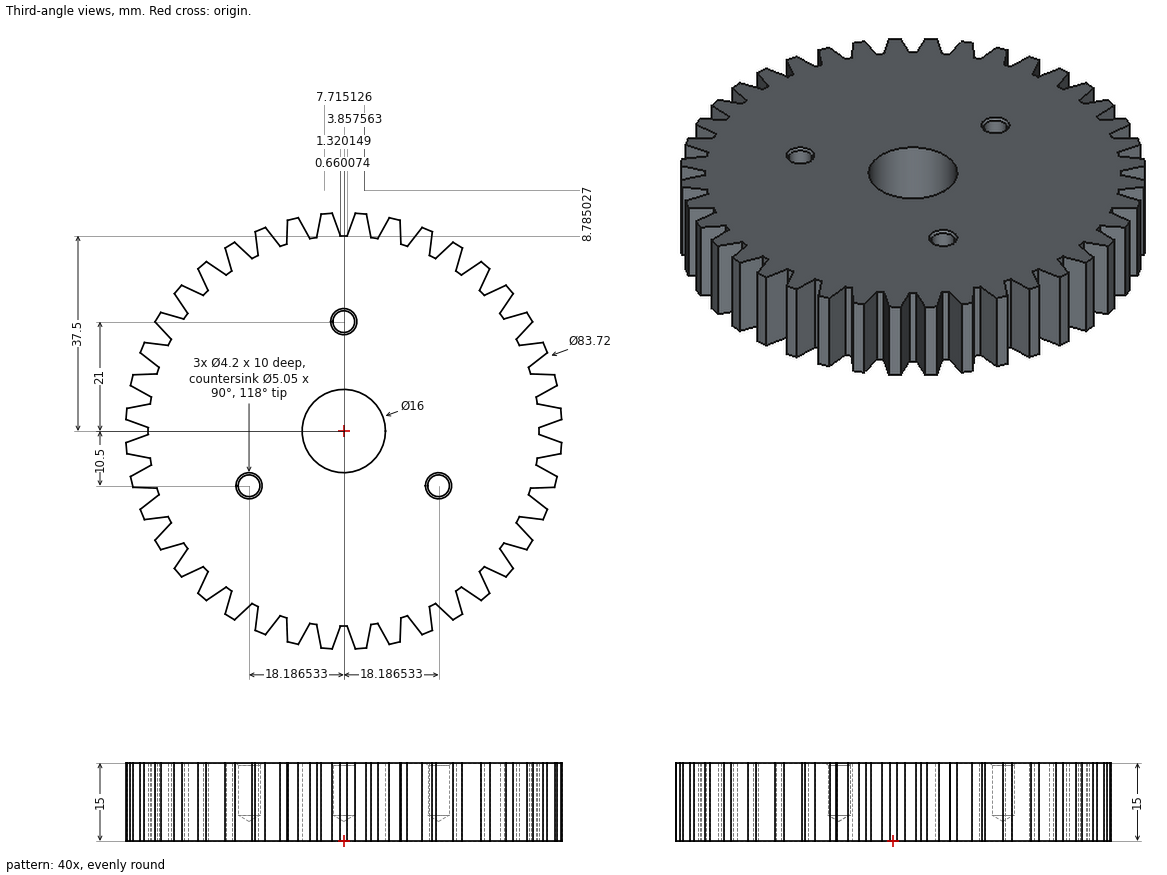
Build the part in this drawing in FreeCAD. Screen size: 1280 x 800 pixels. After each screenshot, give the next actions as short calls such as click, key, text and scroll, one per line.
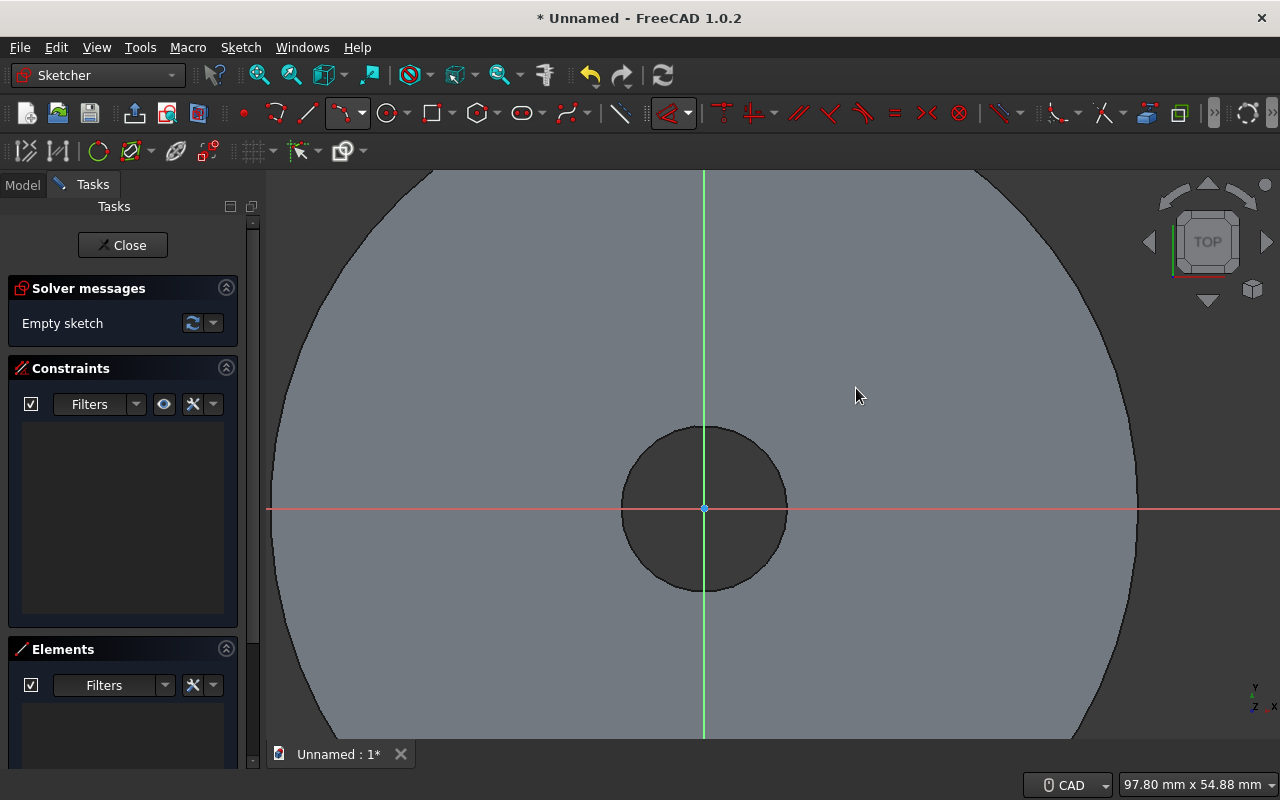
click(388, 114)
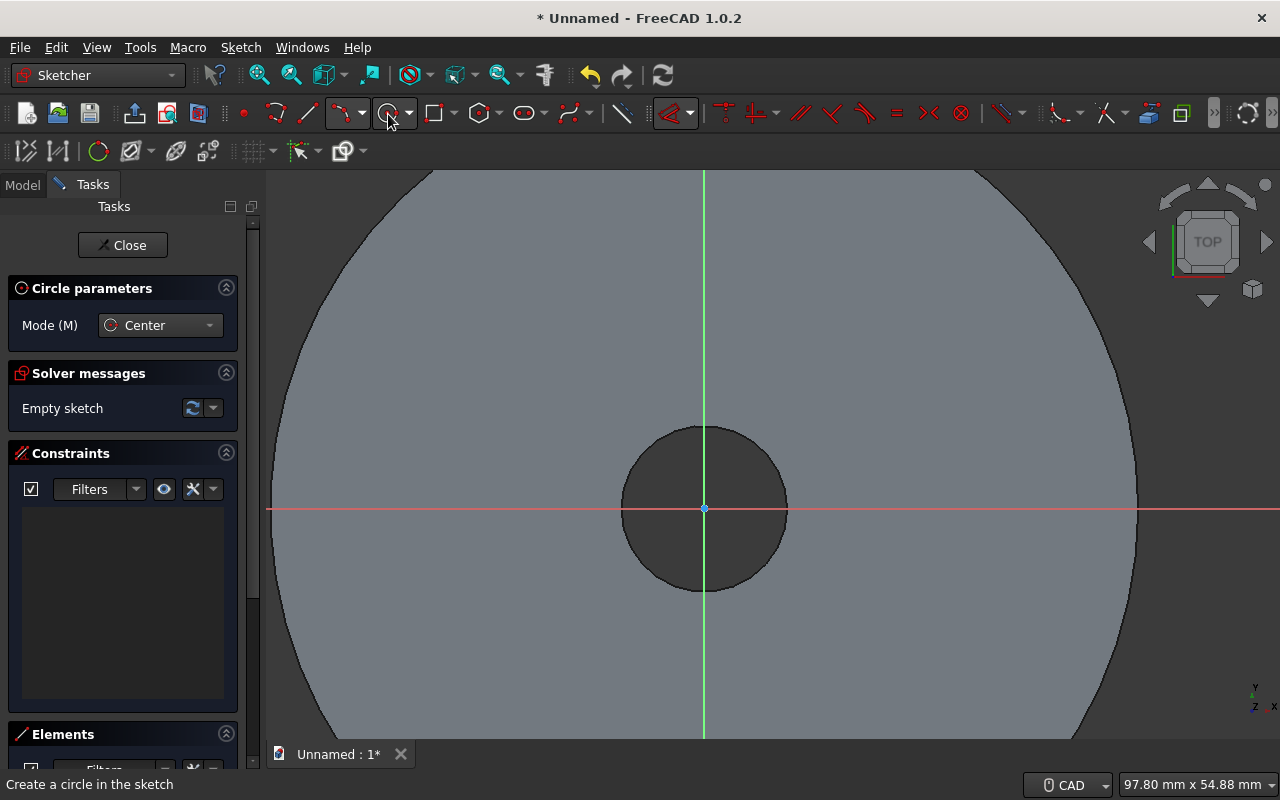
click(516, 618)
click(531, 602)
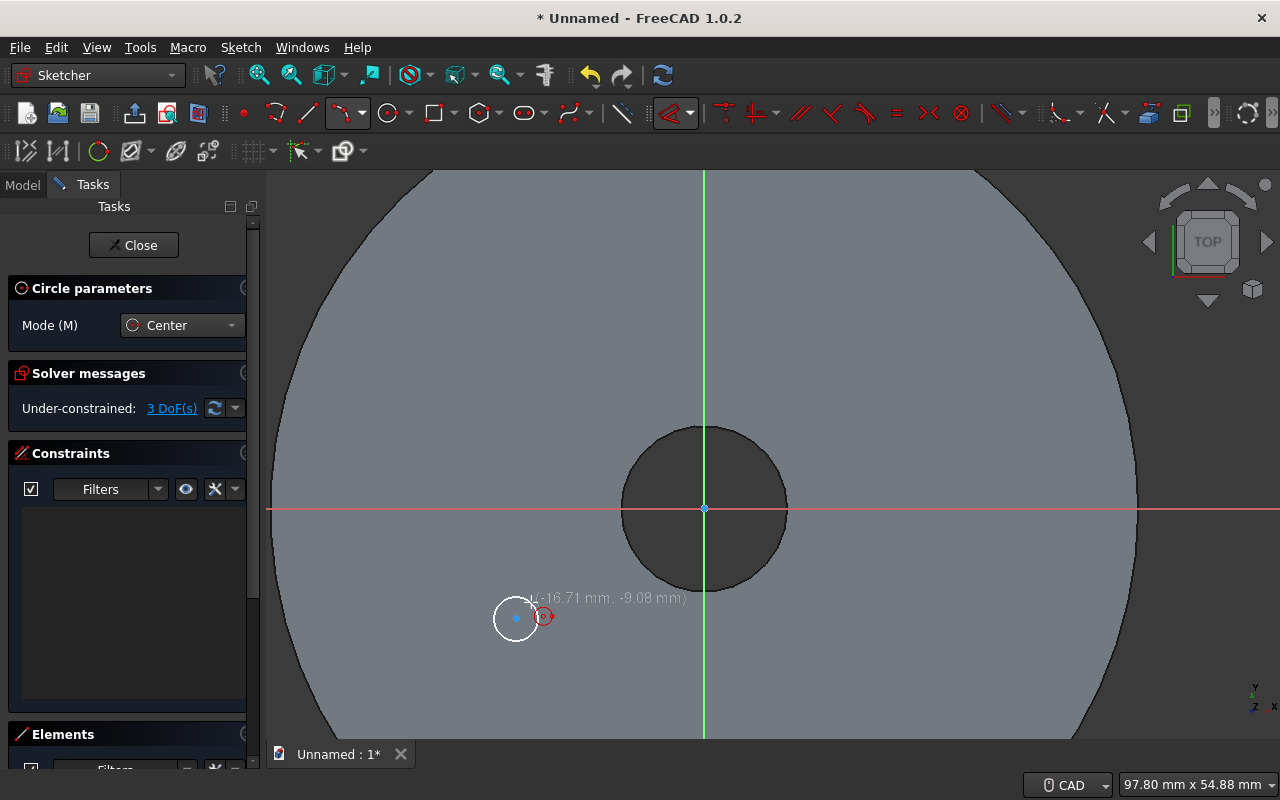
click(704, 291)
click(720, 276)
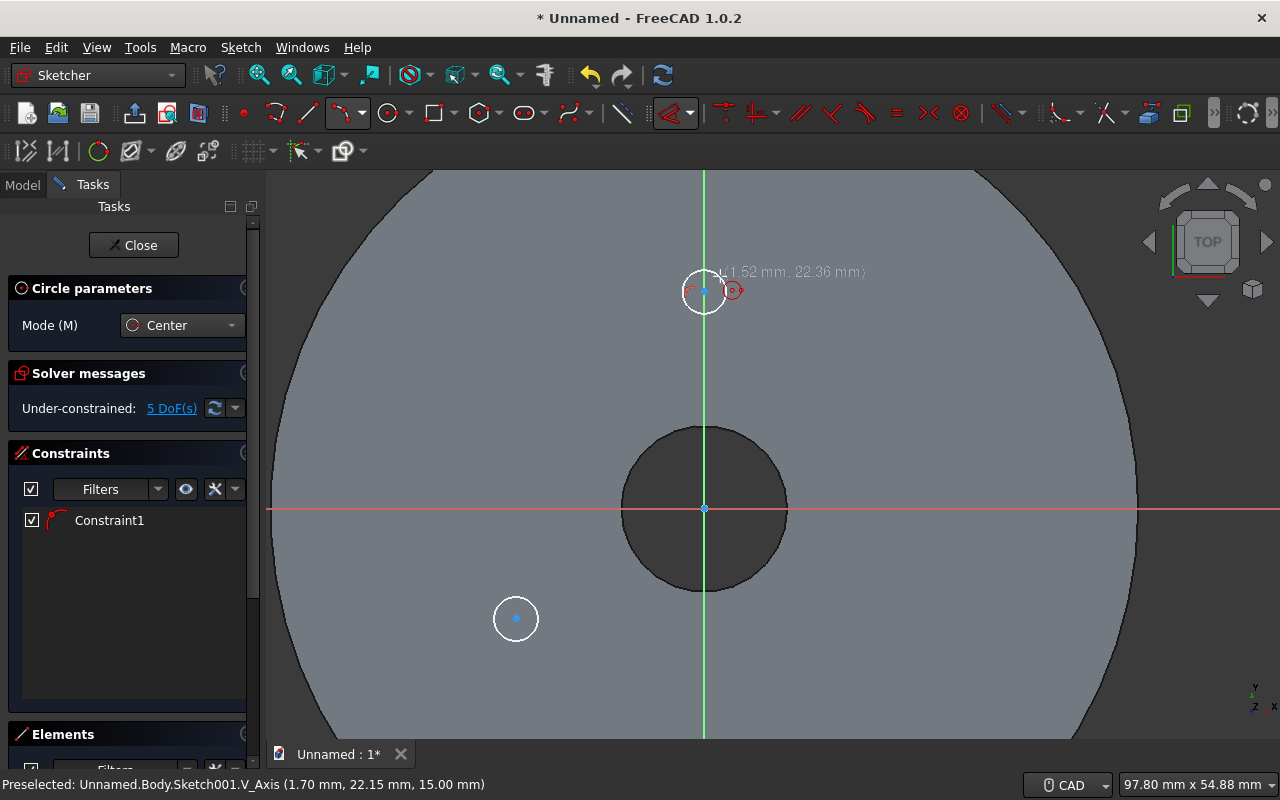
click(893, 618)
click(908, 602)
key(Escape)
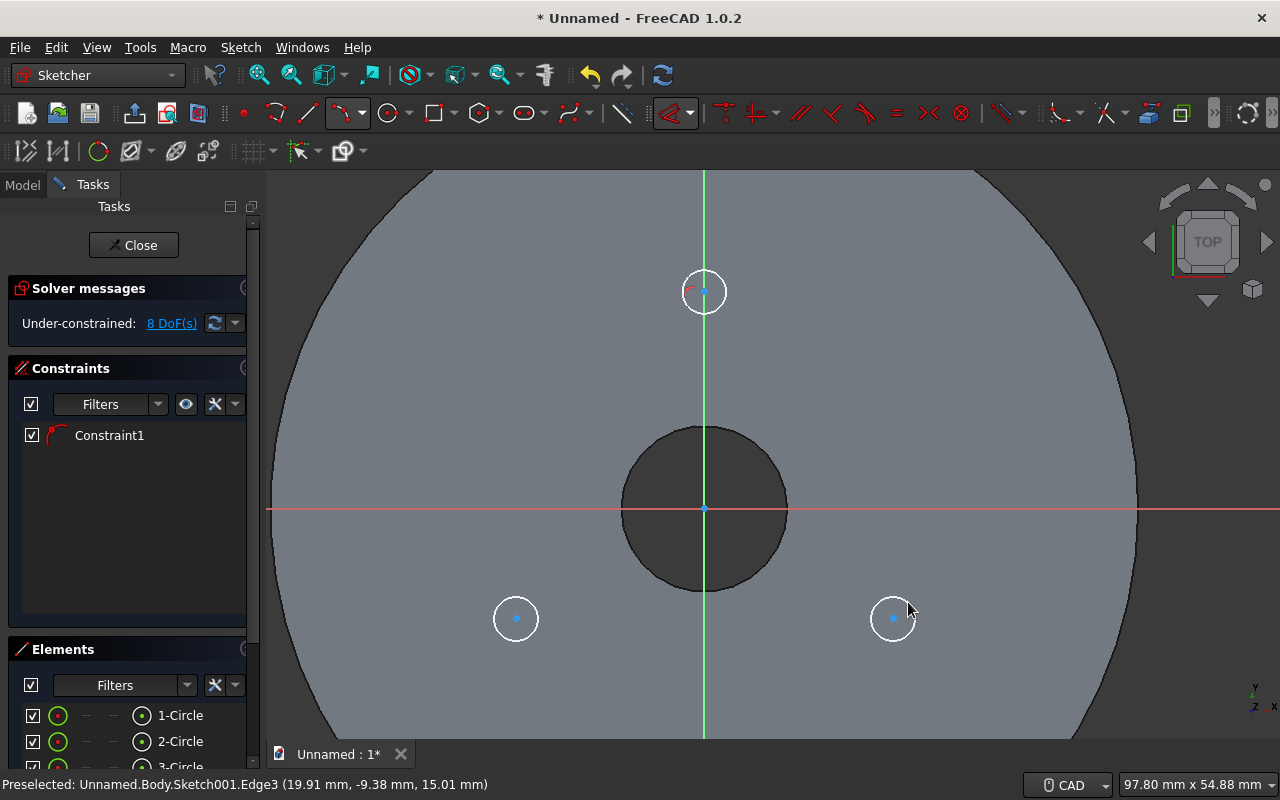
click(531, 603)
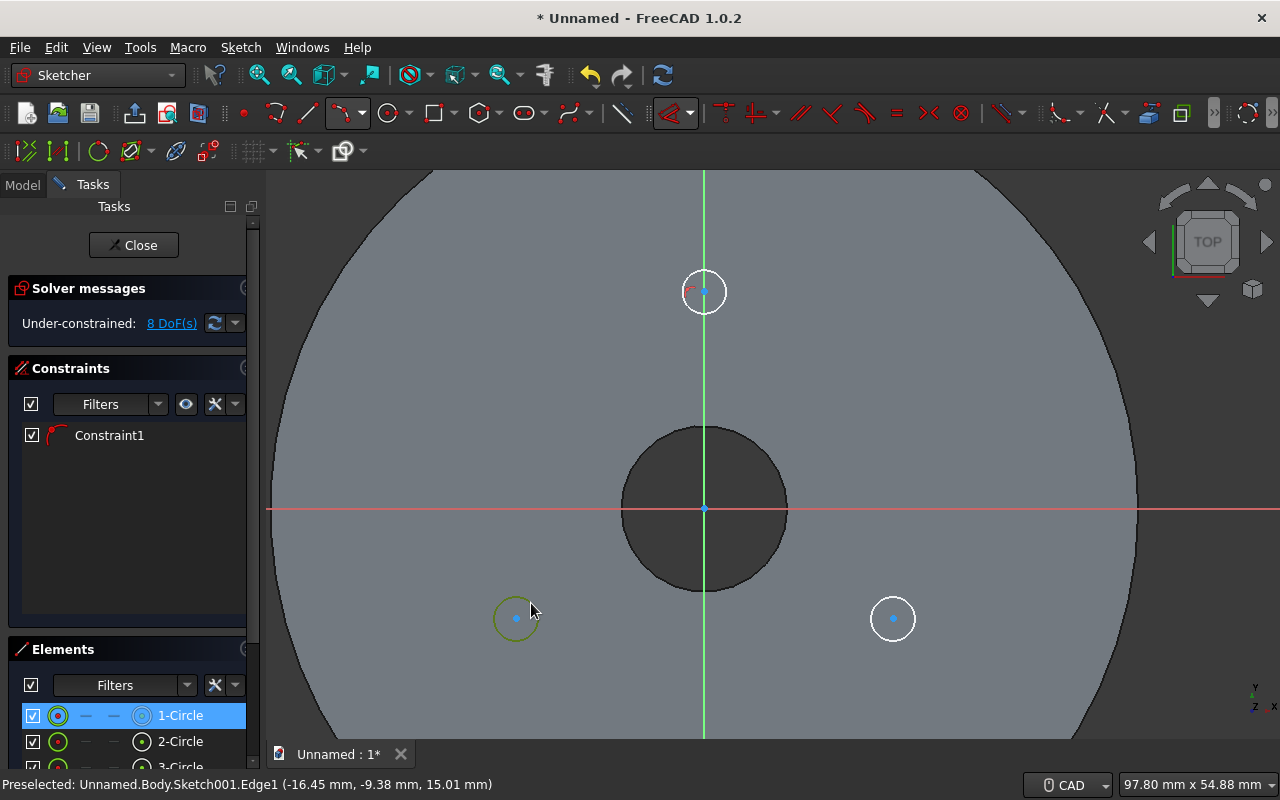
click(720, 277)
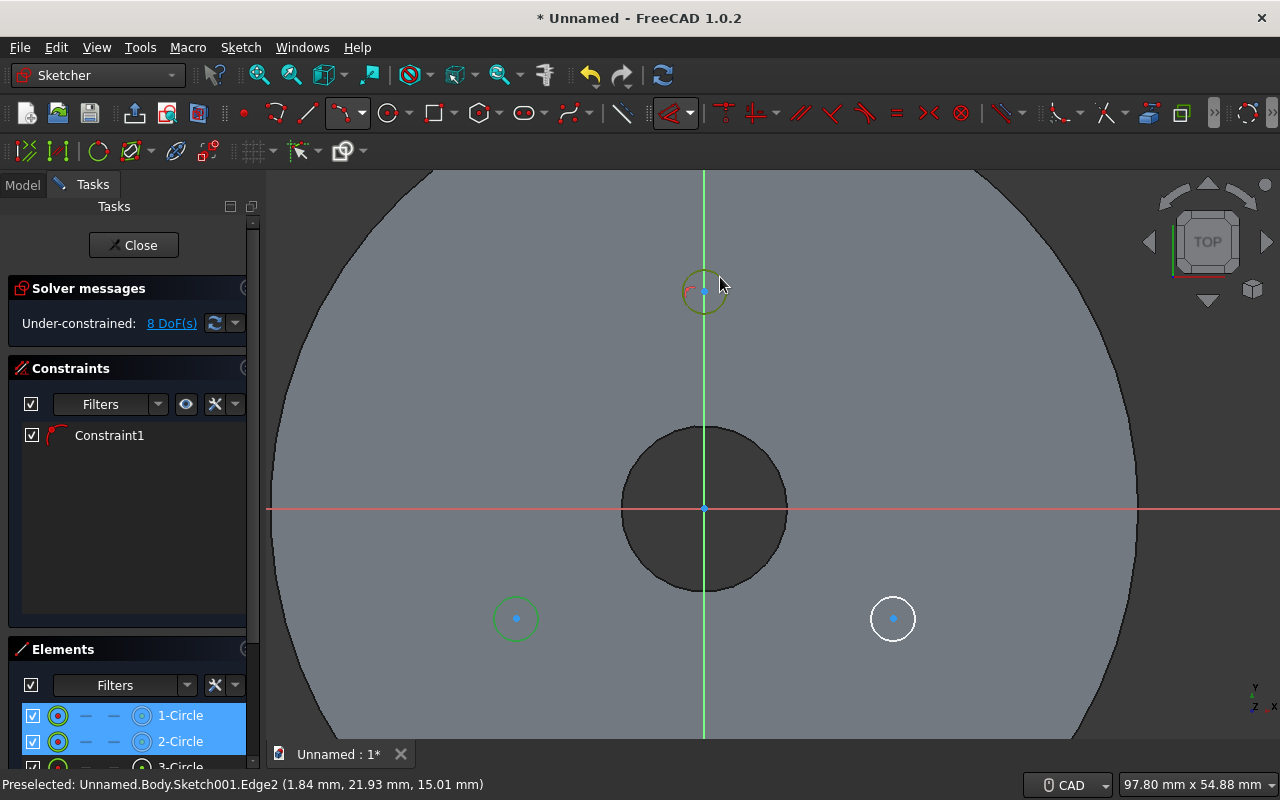
click(908, 603)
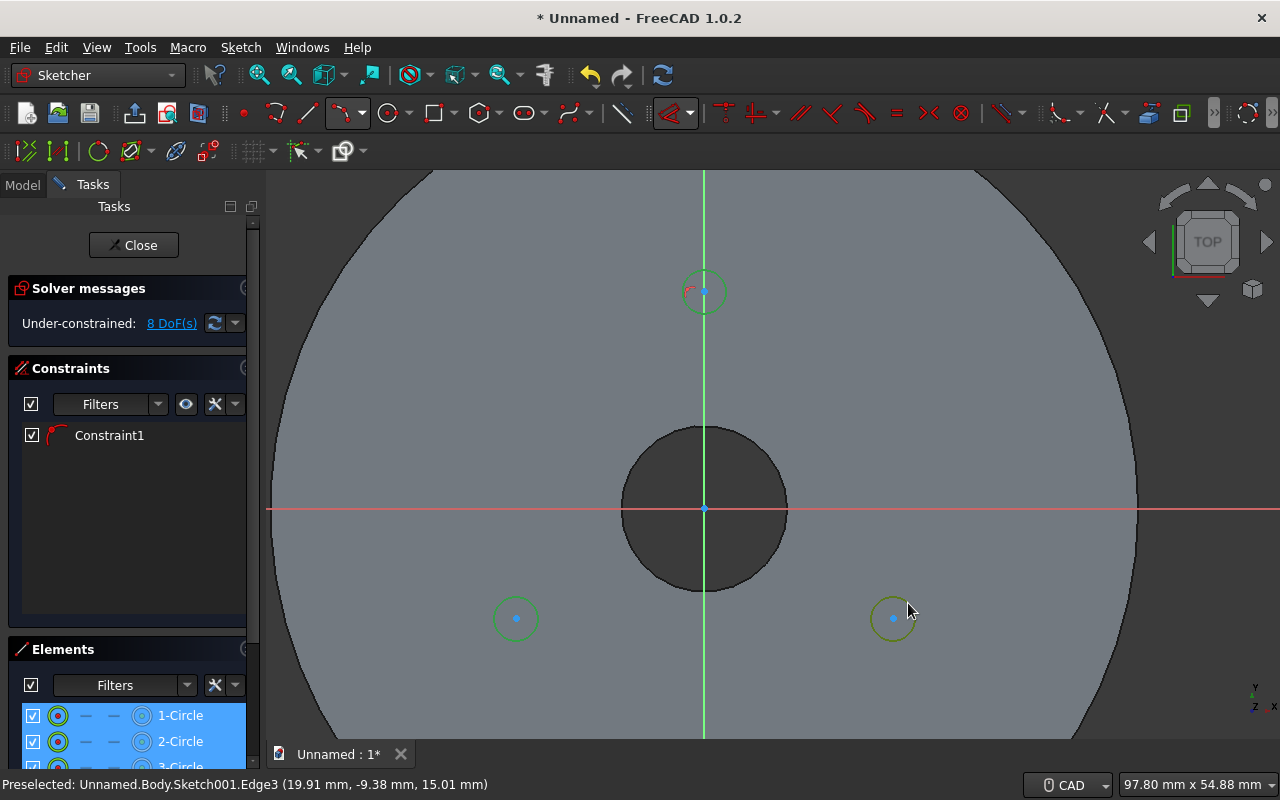
click(898, 114)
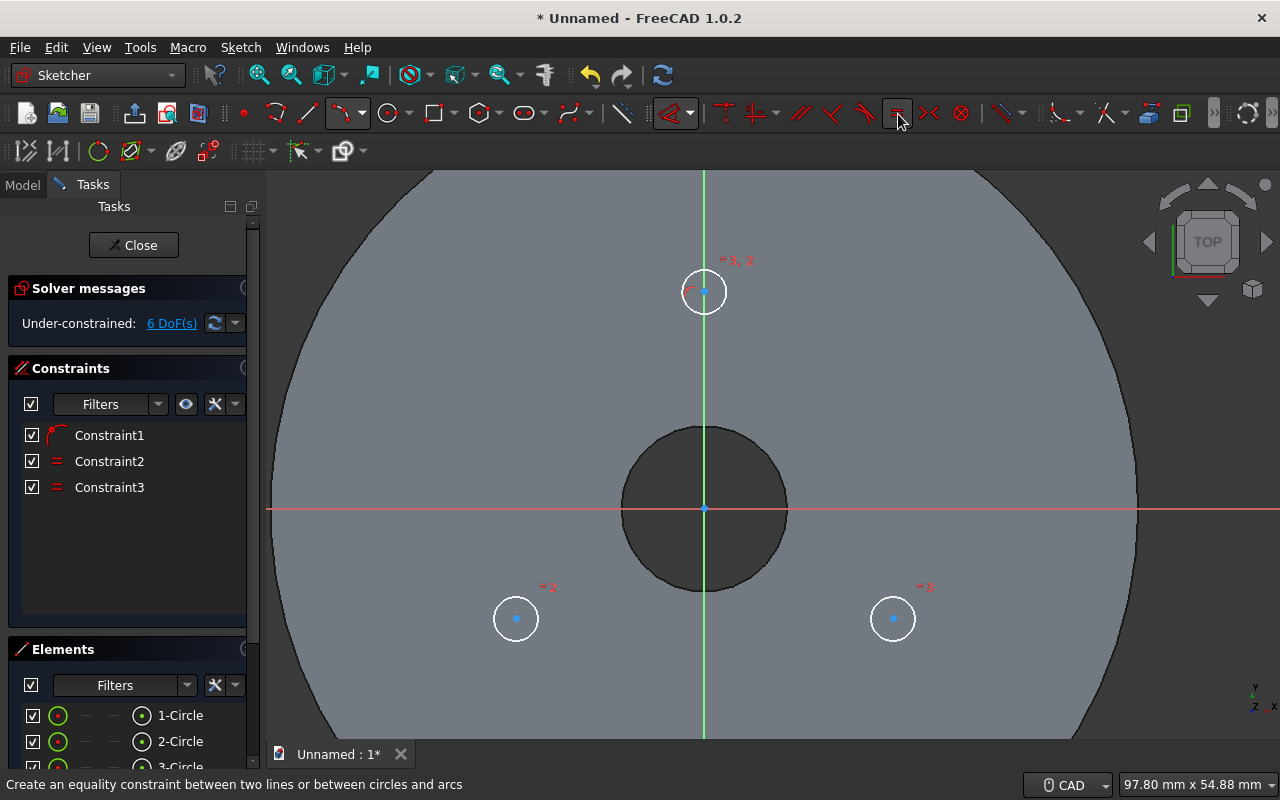
click(516, 619)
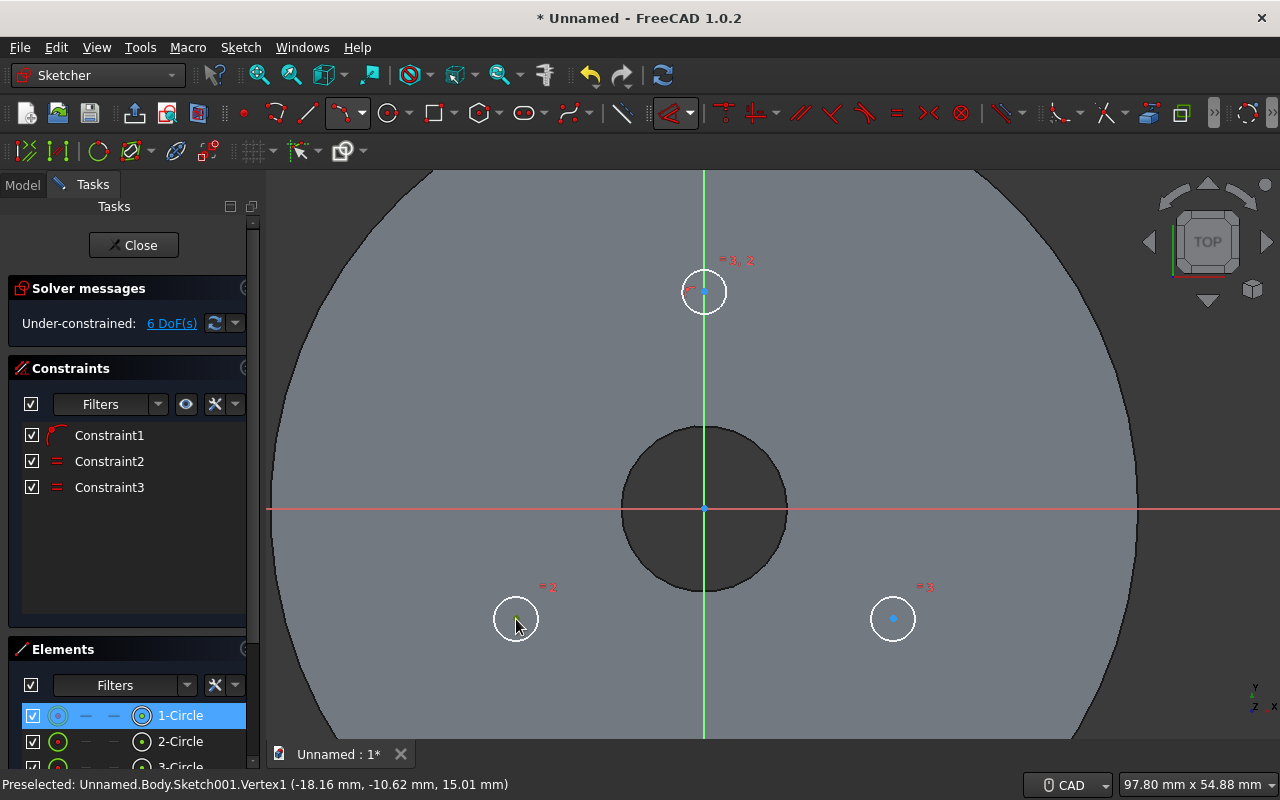
click(893, 619)